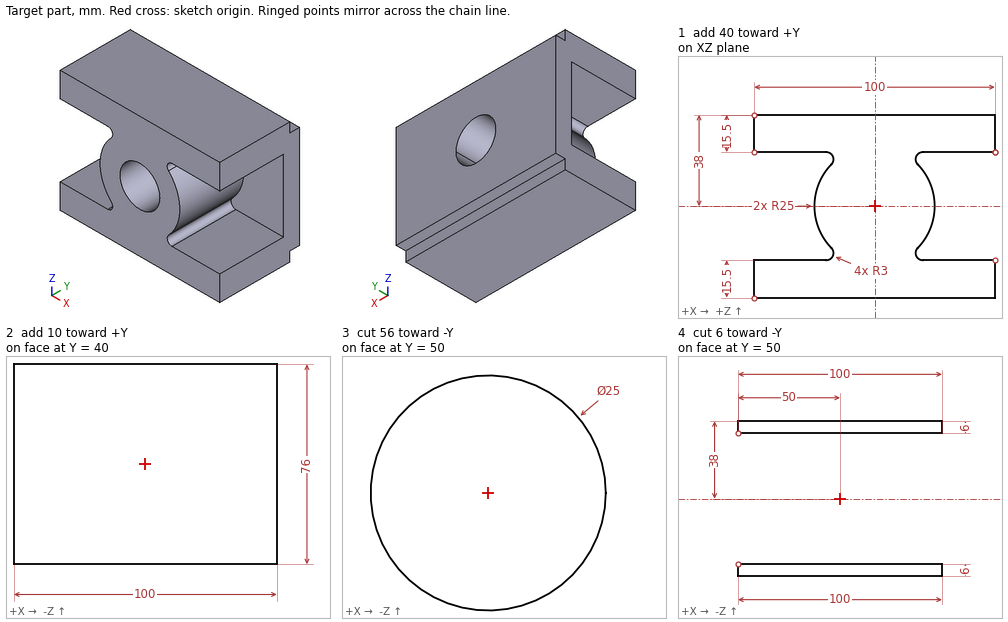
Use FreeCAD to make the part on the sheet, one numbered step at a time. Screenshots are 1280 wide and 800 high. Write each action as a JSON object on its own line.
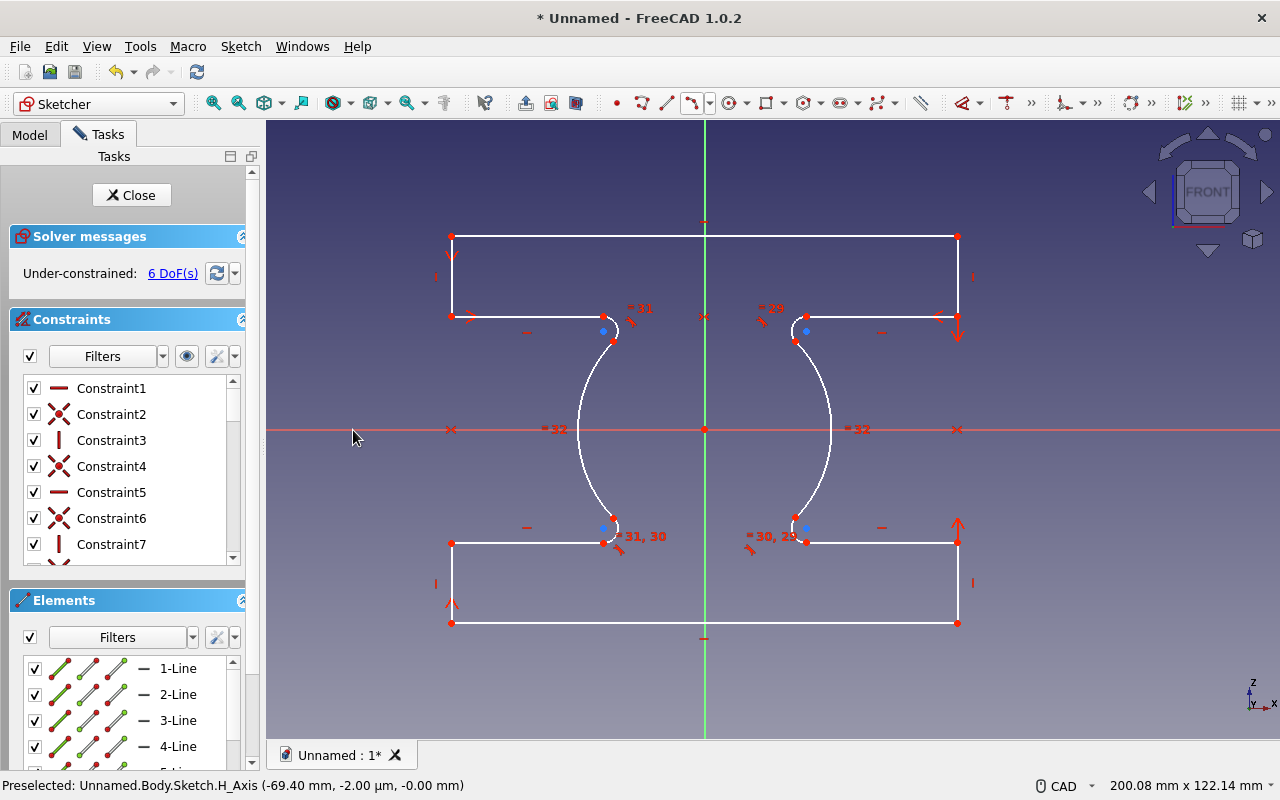
{"action": "left_click", "coordinate": [962, 104]}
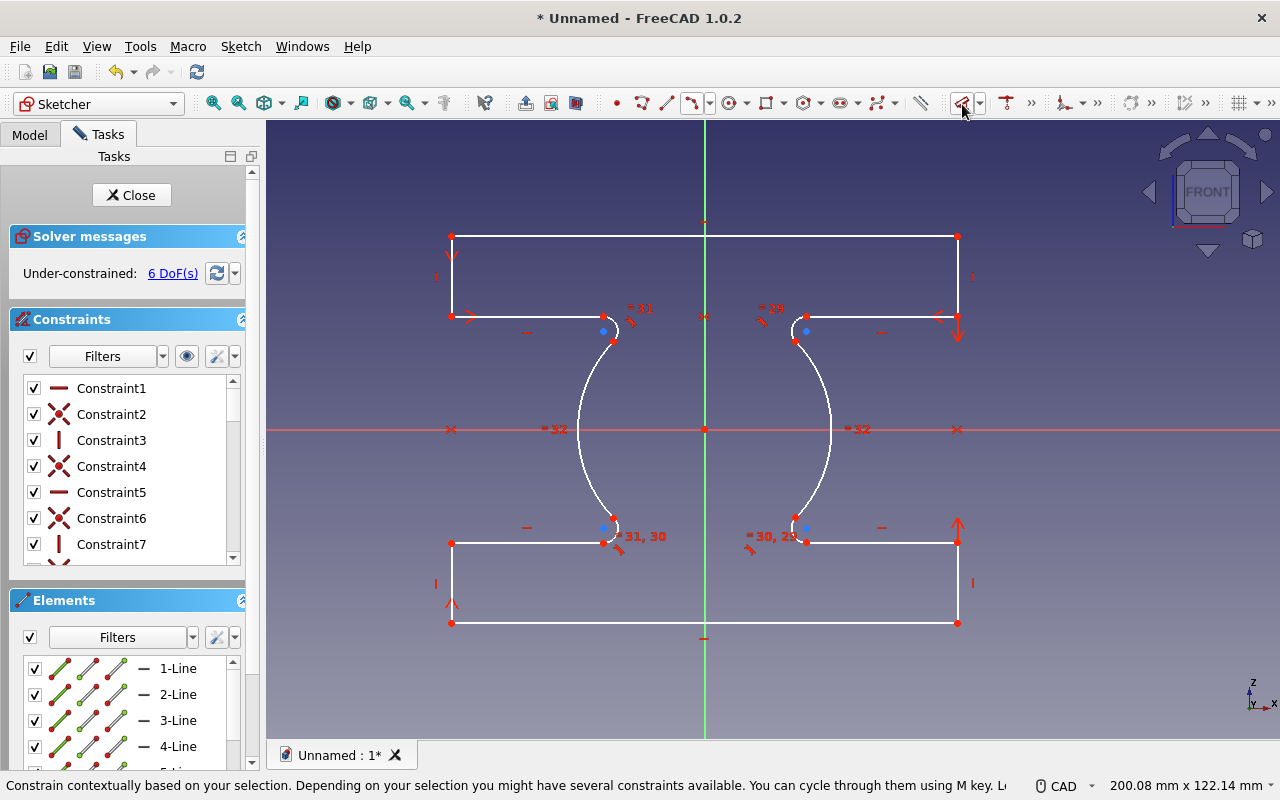
{"action": "scroll", "coordinate": [797, 320], "scroll_direction": "up", "scroll_amount": 5}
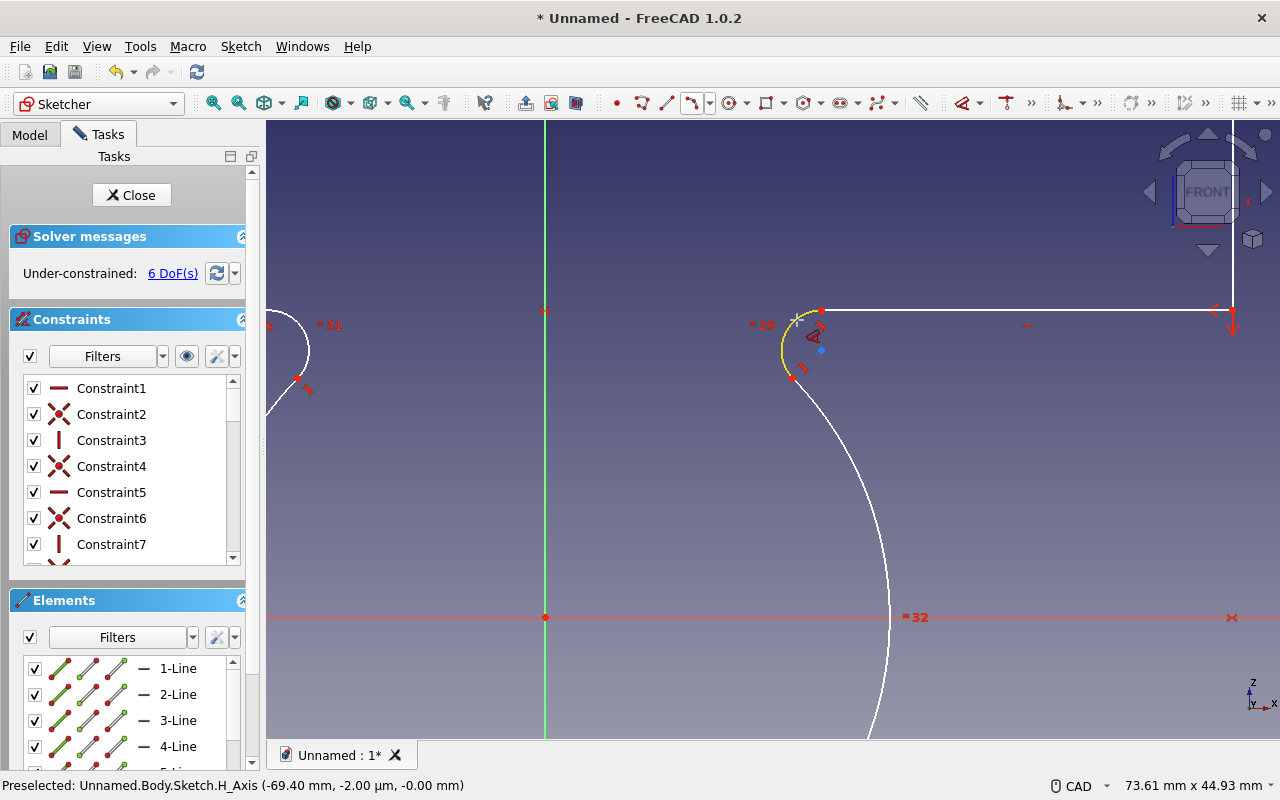
{"action": "left_click", "coordinate": [796, 320]}
{"action": "left_click", "coordinate": [775, 296]}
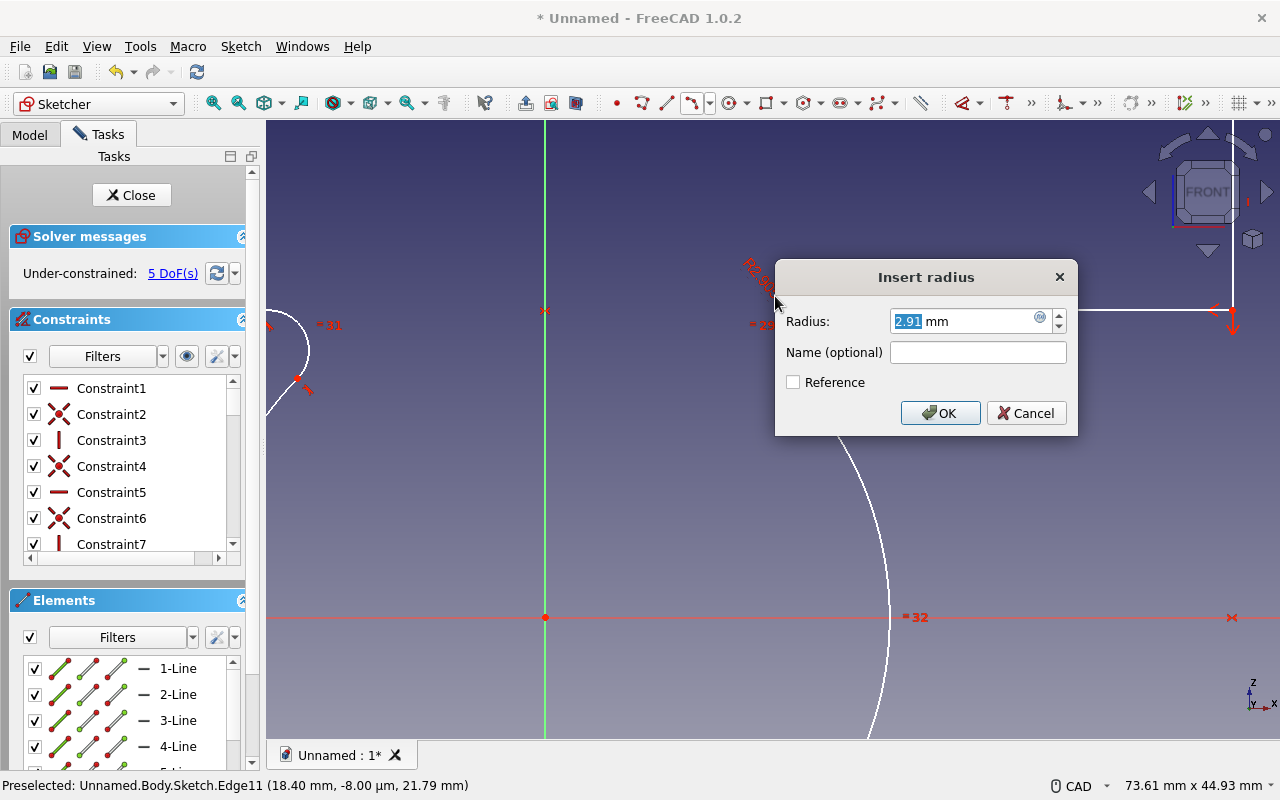
{"action": "type", "text": "3"}
{"action": "key", "text": "Return"}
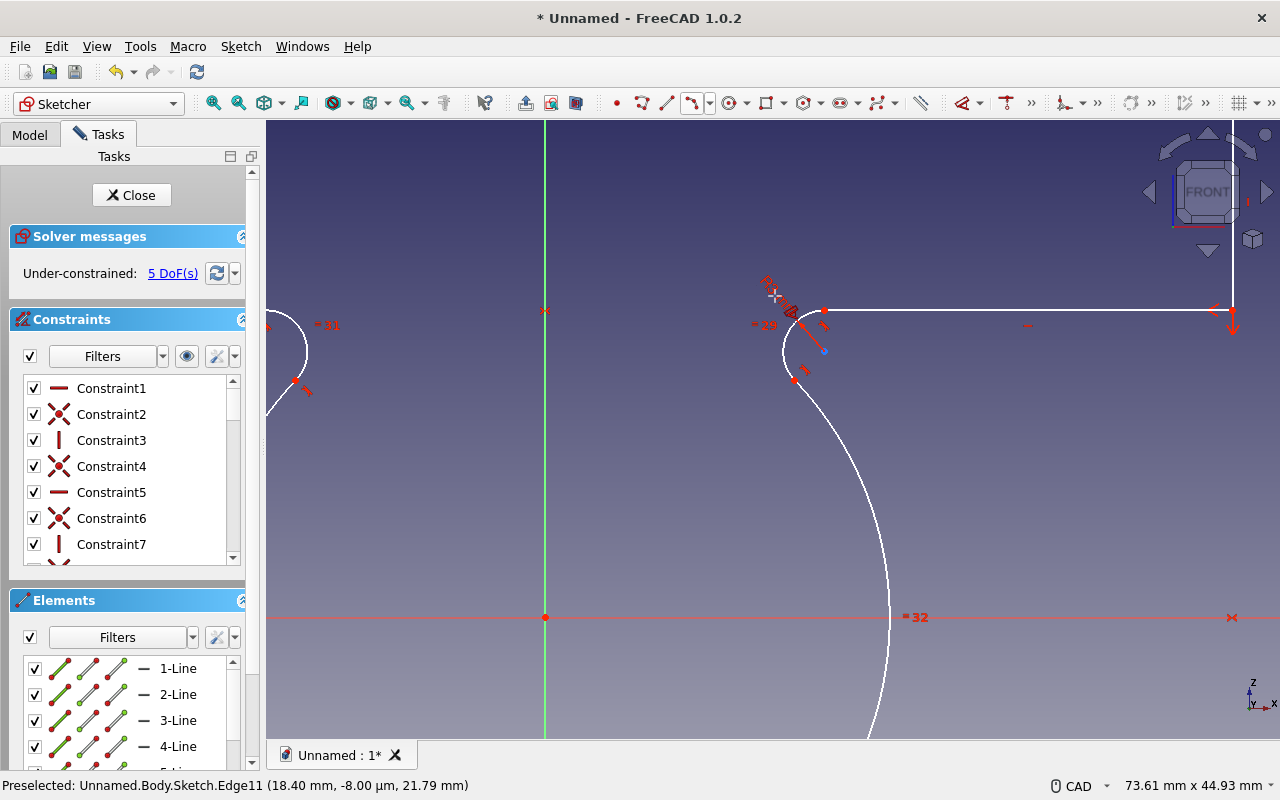
{"action": "left_click", "coordinate": [874, 515]}
{"action": "left_click", "coordinate": [905, 505]}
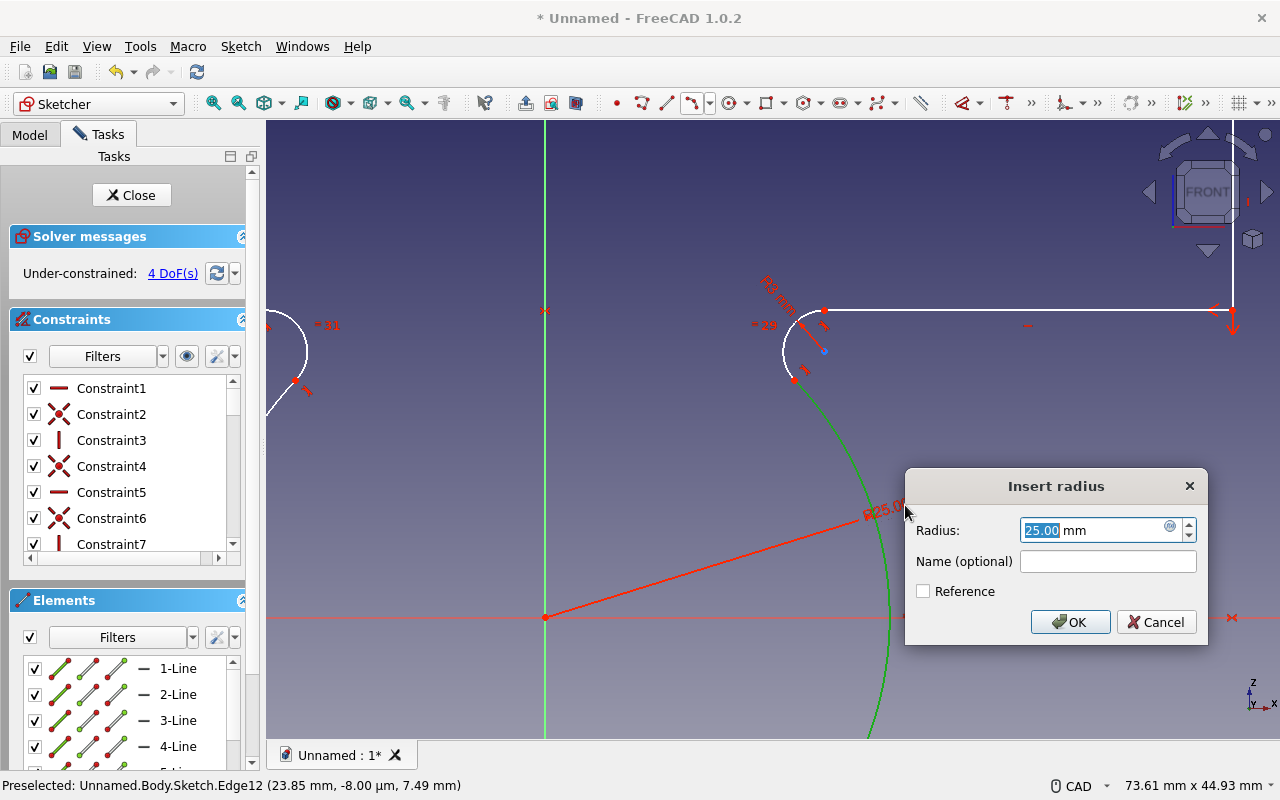
{"action": "type", "text": "25"}
{"action": "key", "text": "Return"}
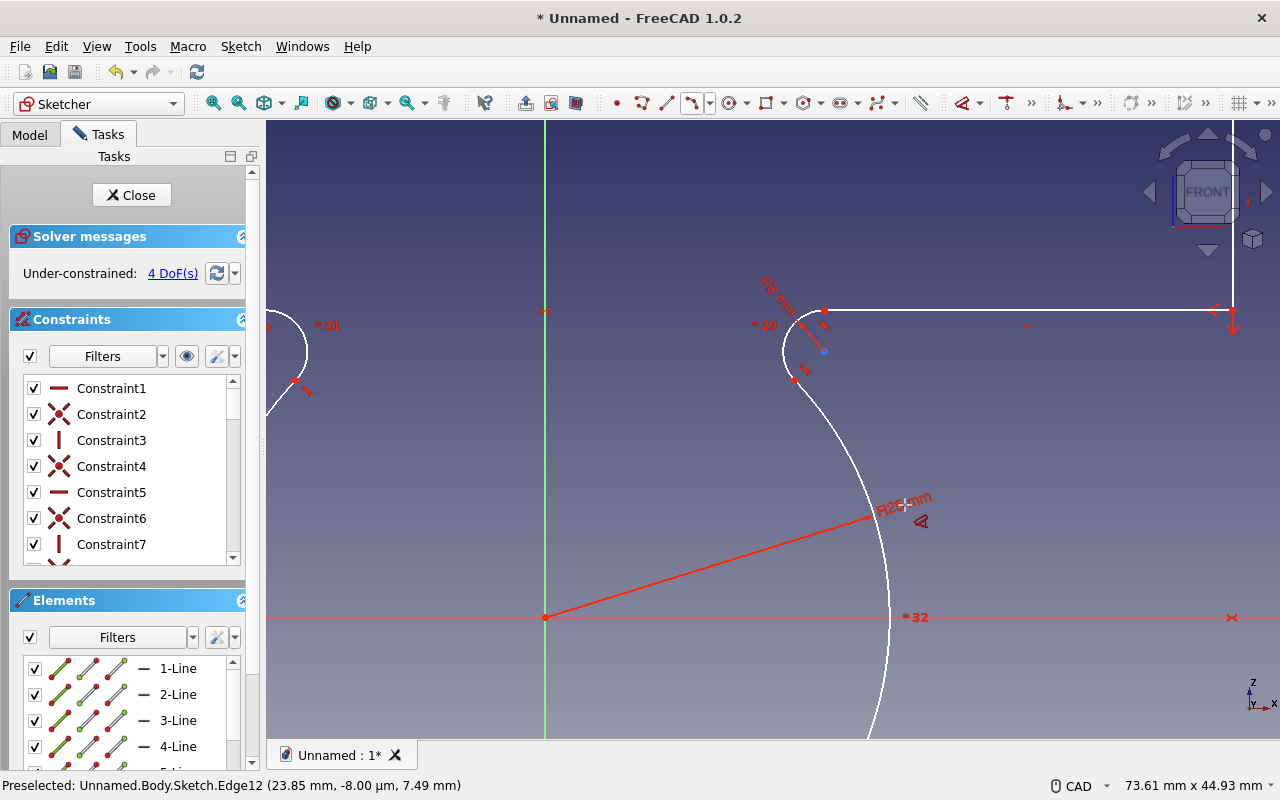
{"action": "scroll", "coordinate": [797, 320], "scroll_direction": "down", "scroll_amount": 5}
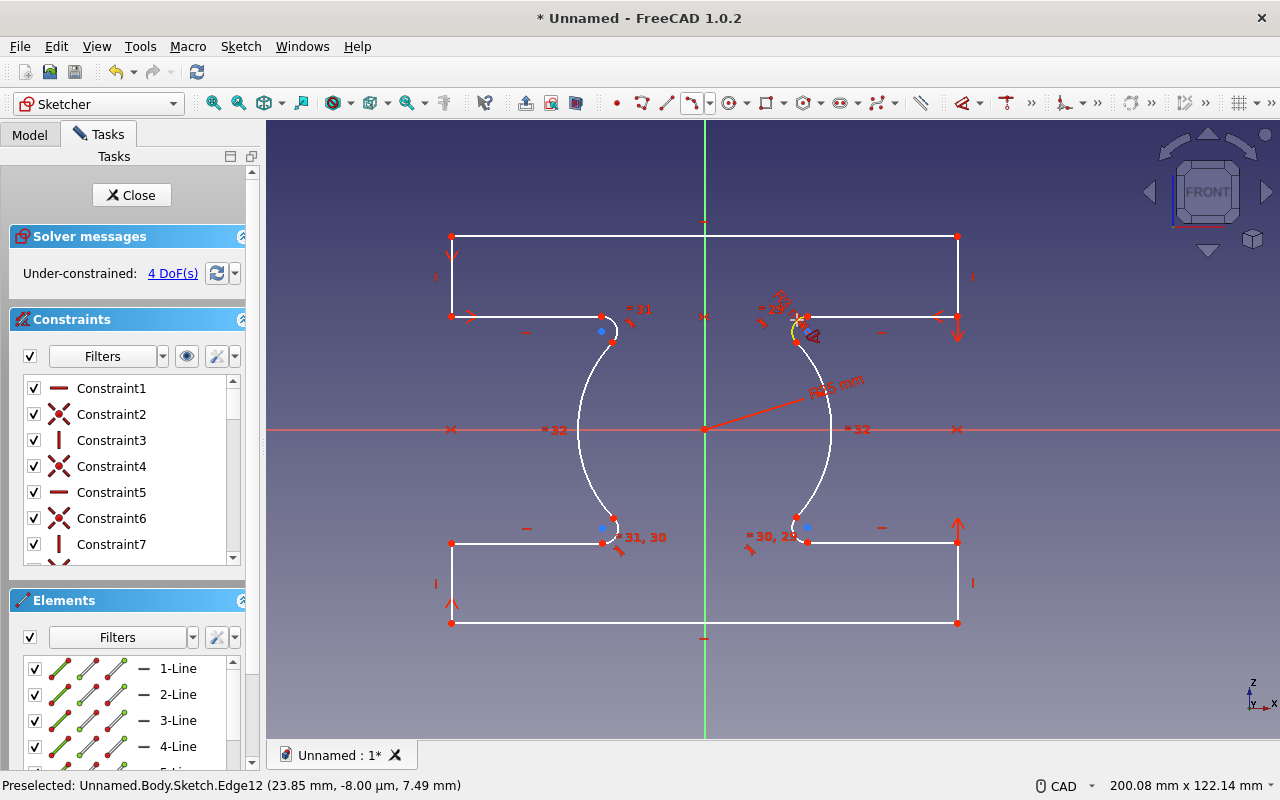
{"action": "left_click", "coordinate": [604, 236]}
{"action": "left_click", "coordinate": [588, 202]}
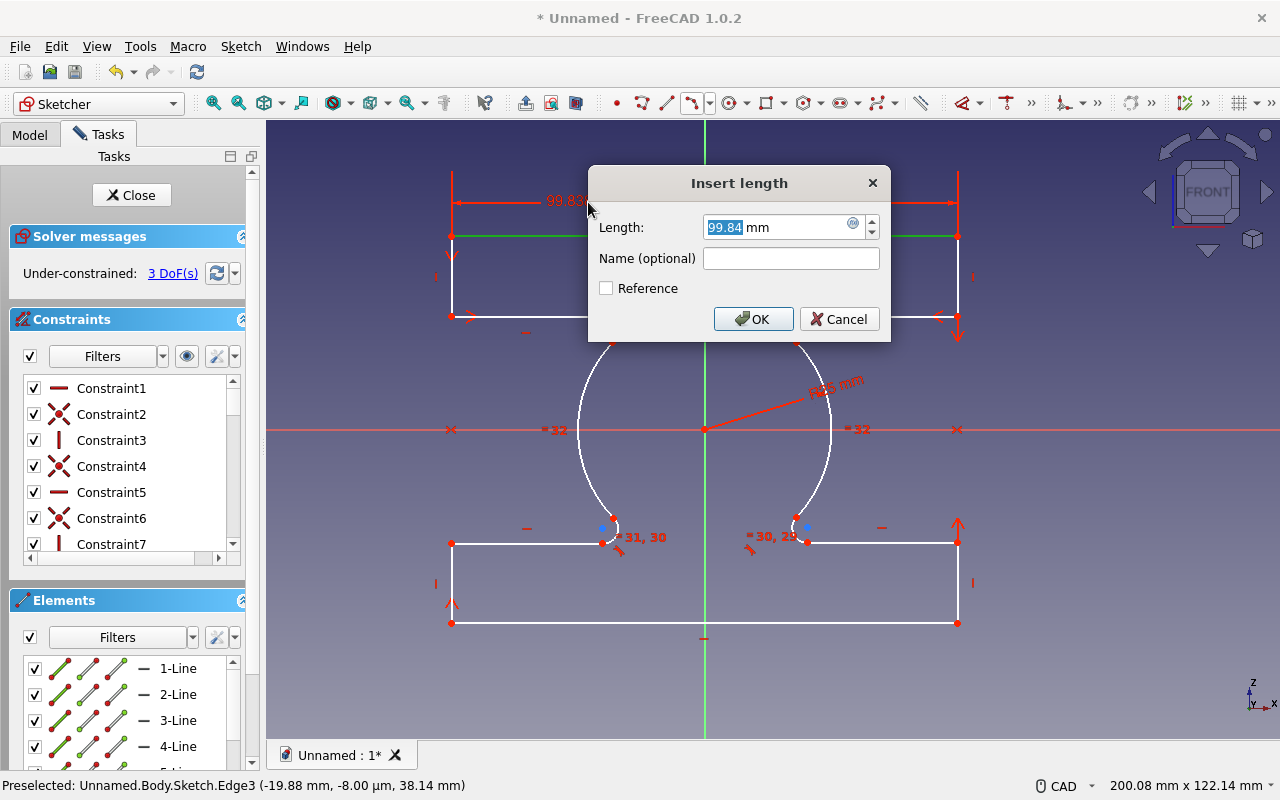
{"action": "type", "text": "100"}
{"action": "key", "text": "Return"}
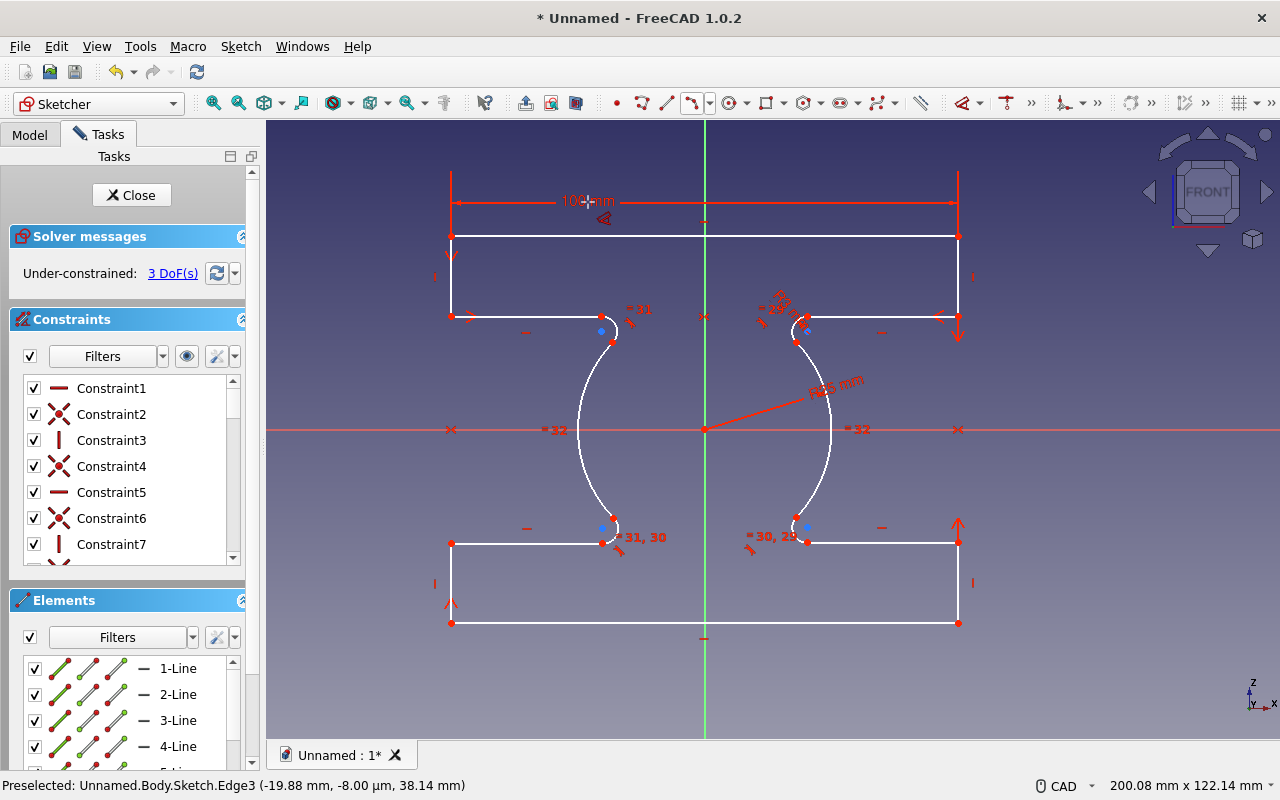
{"action": "left_click", "coordinate": [451, 236]}
{"action": "left_click", "coordinate": [417, 333]}